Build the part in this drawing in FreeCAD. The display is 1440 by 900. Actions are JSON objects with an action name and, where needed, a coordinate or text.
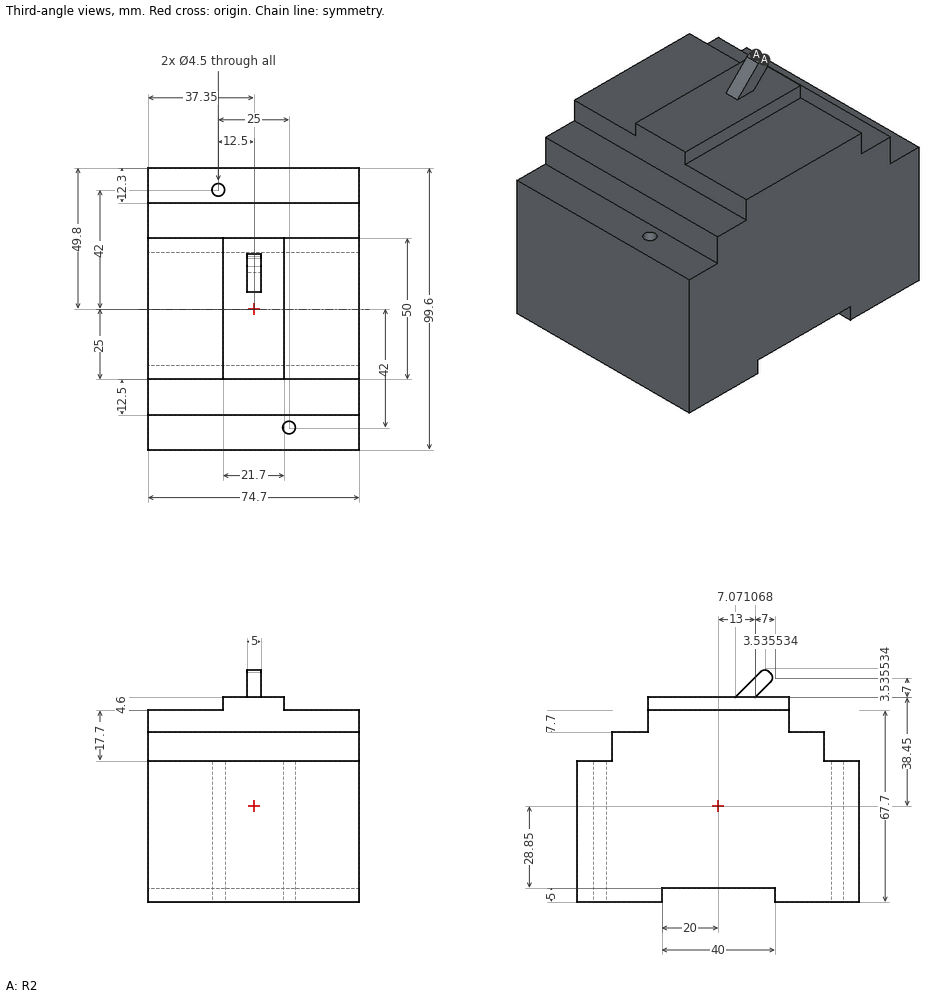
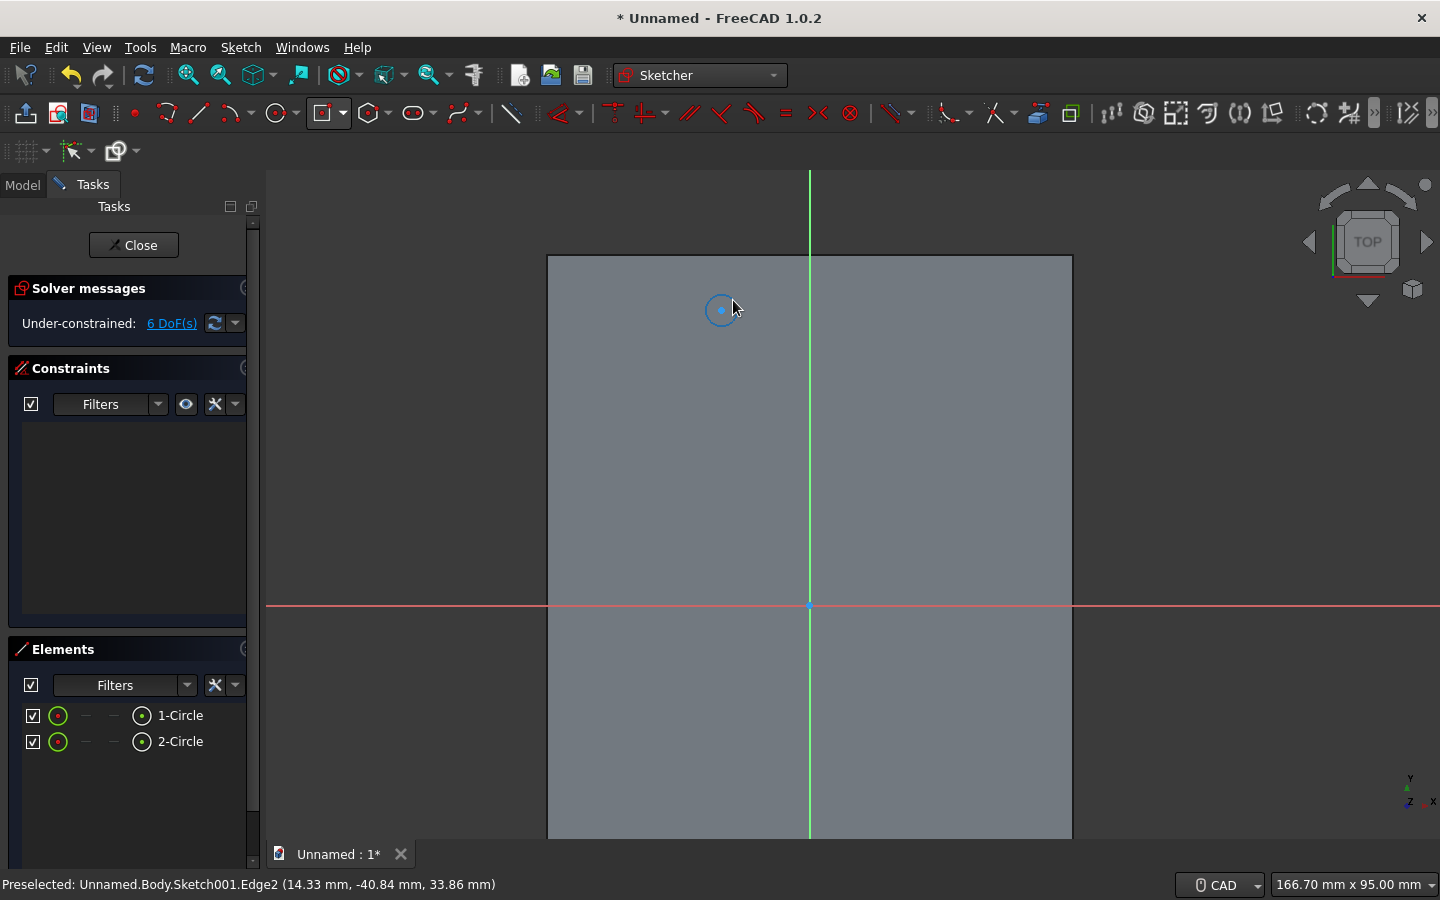
{"action": "left_click", "coordinate": [733, 299]}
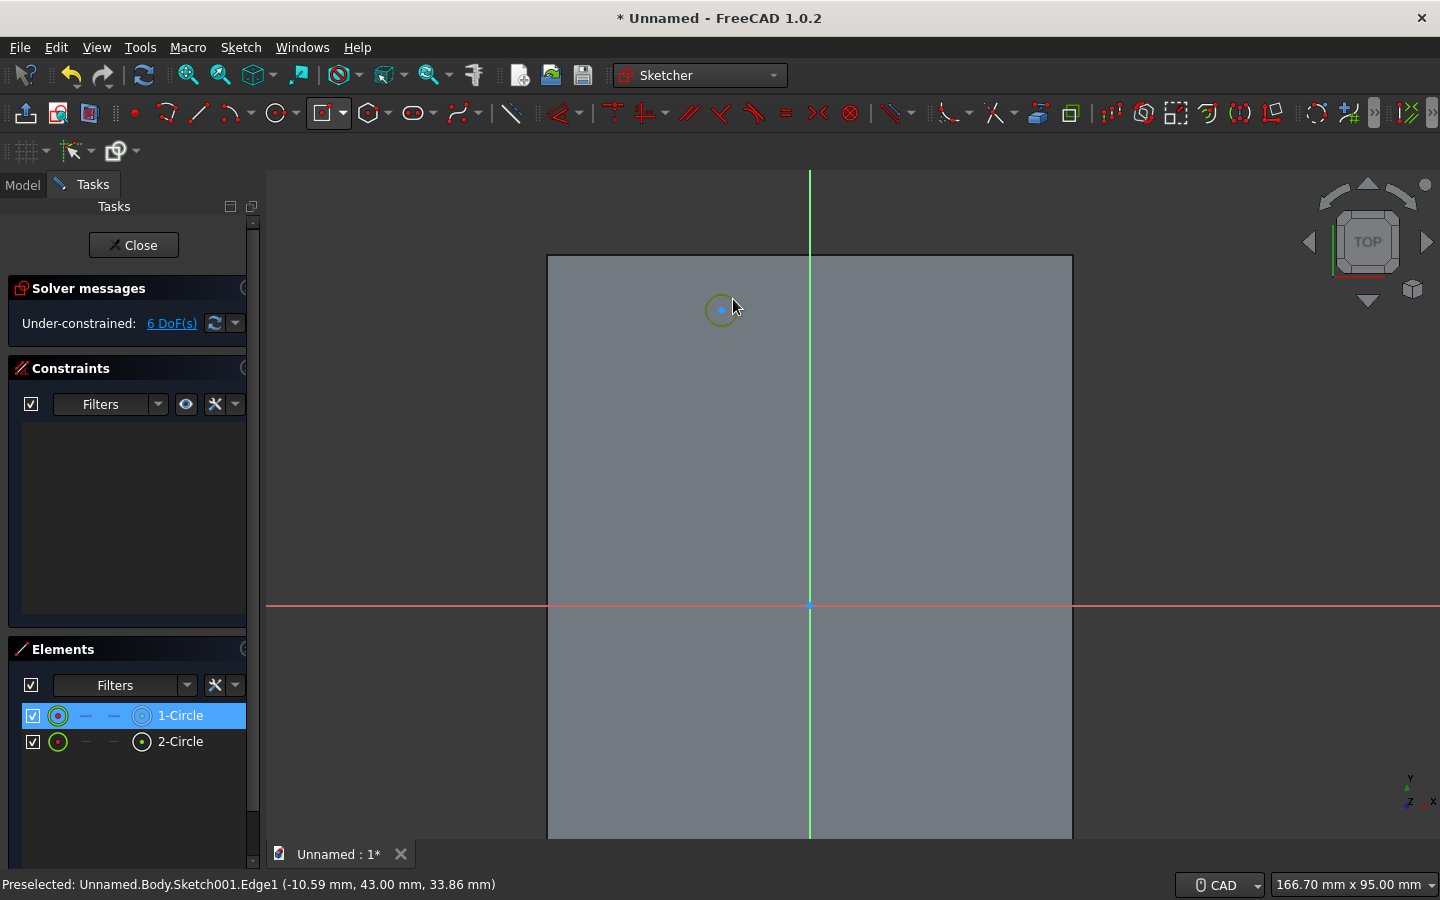
{"action": "scroll", "coordinate": [733, 299], "scroll_direction": "down", "scroll_amount": 2}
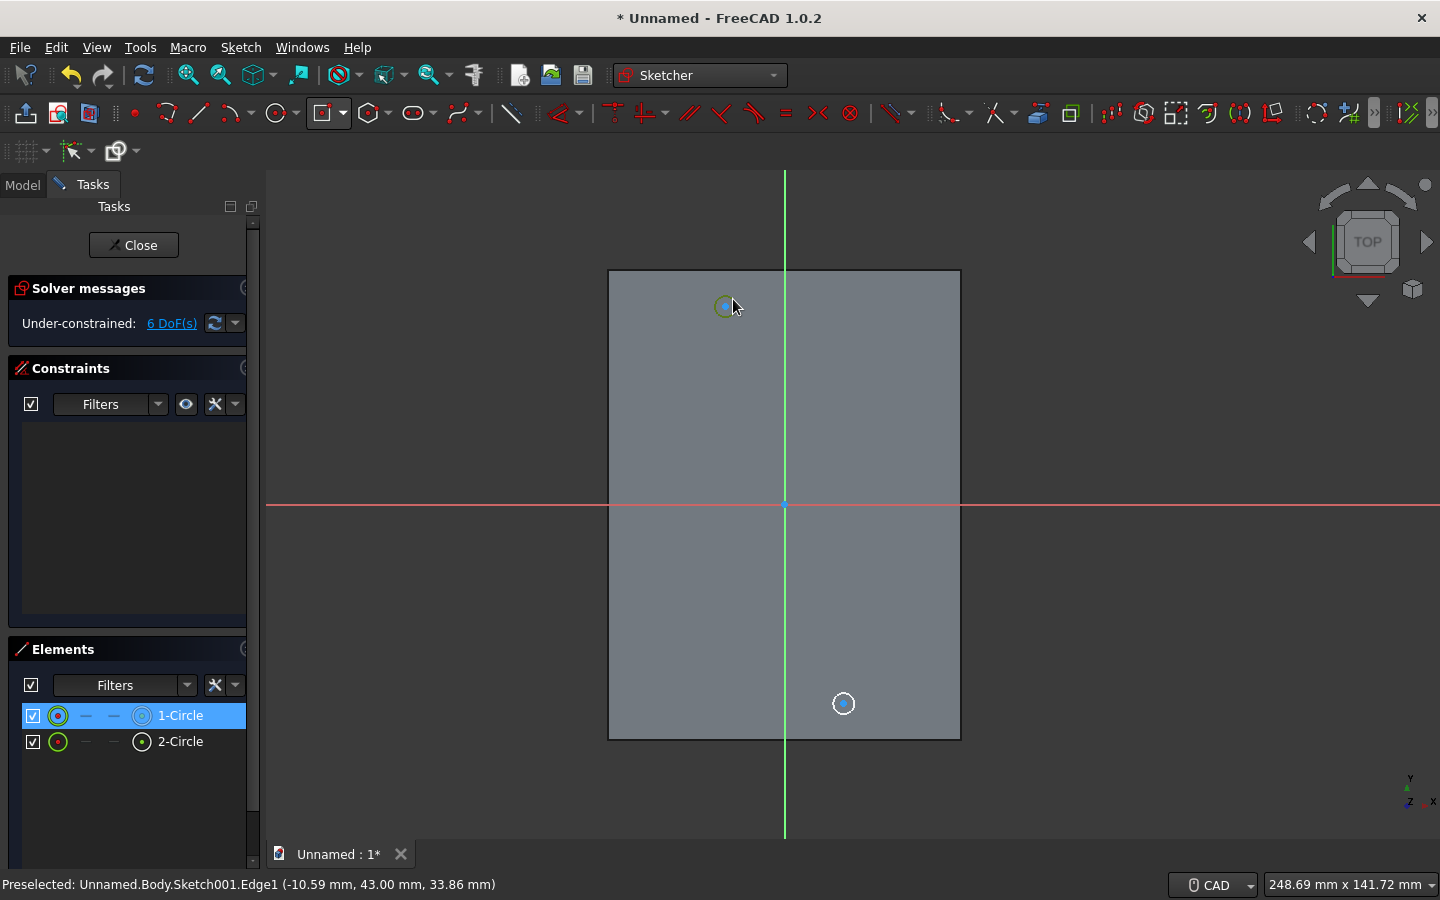
{"action": "scroll", "coordinate": [851, 696], "scroll_direction": "up", "scroll_amount": 2}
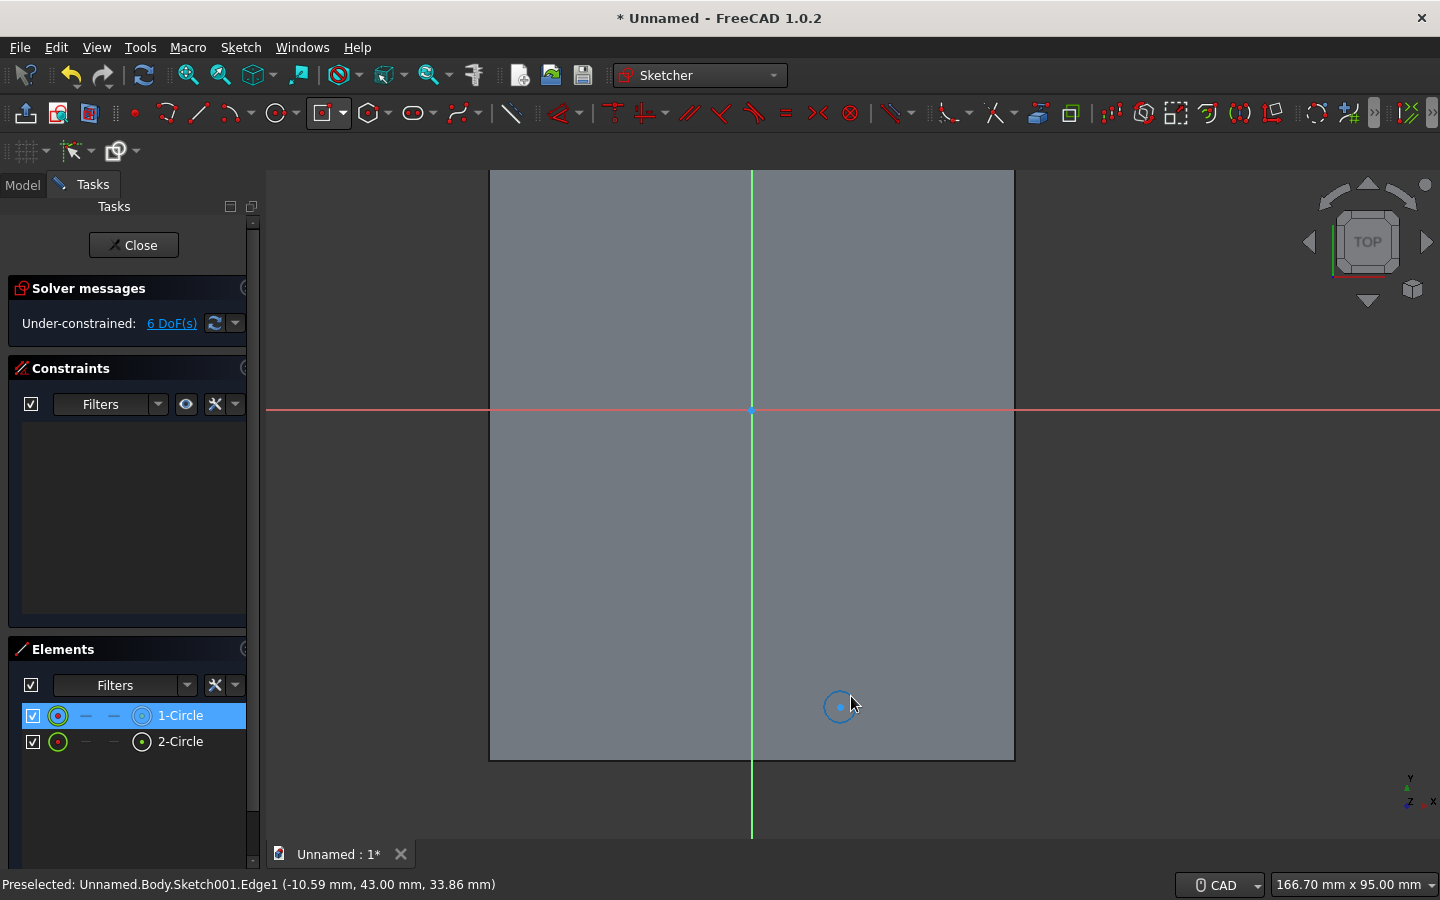
{"action": "left_click", "coordinate": [851, 696]}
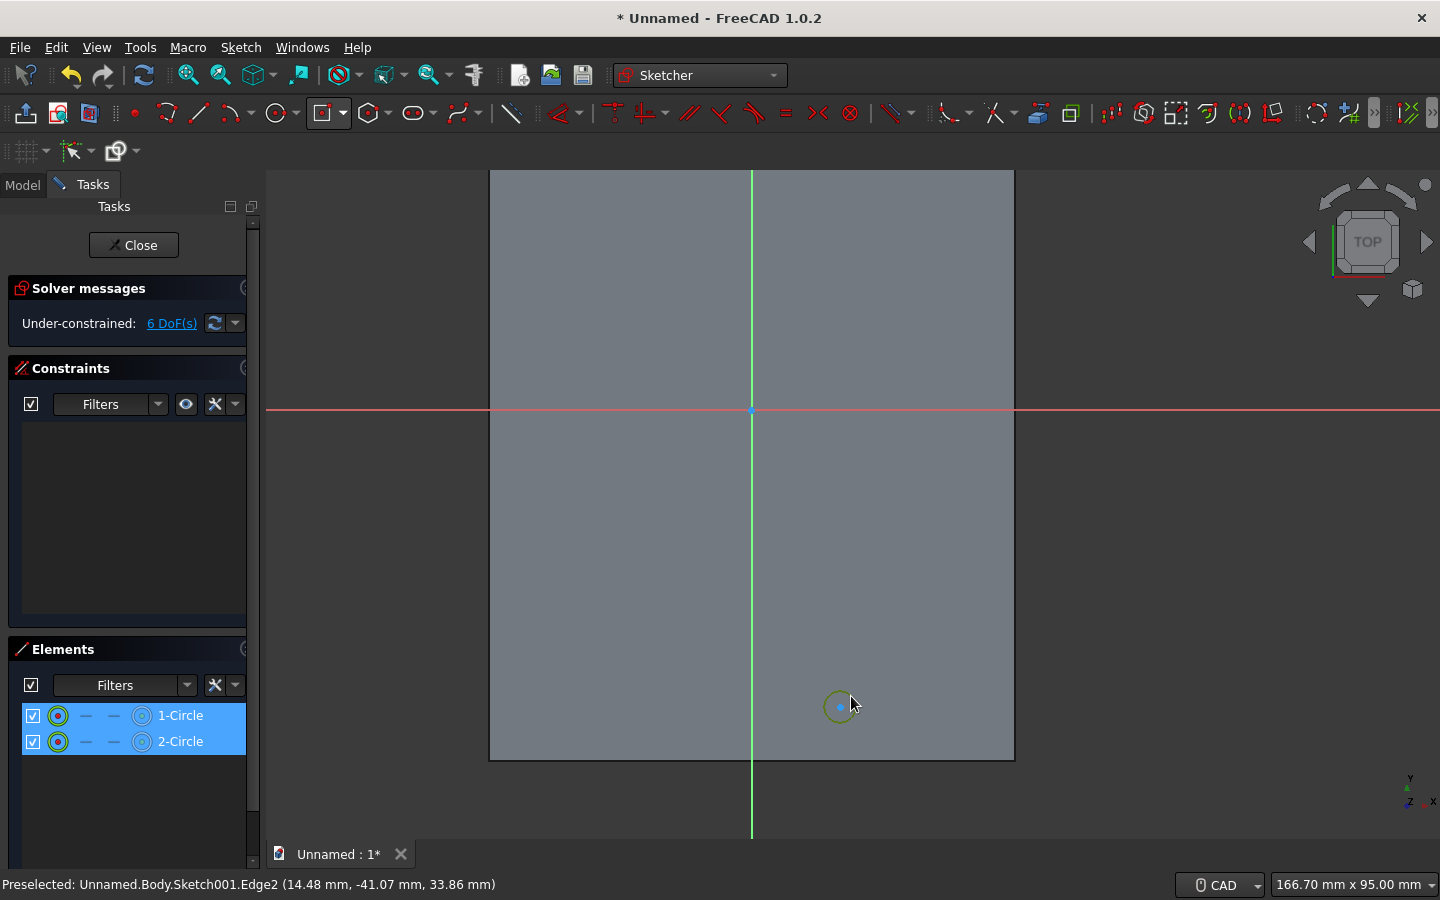
{"action": "left_click", "coordinate": [786, 114]}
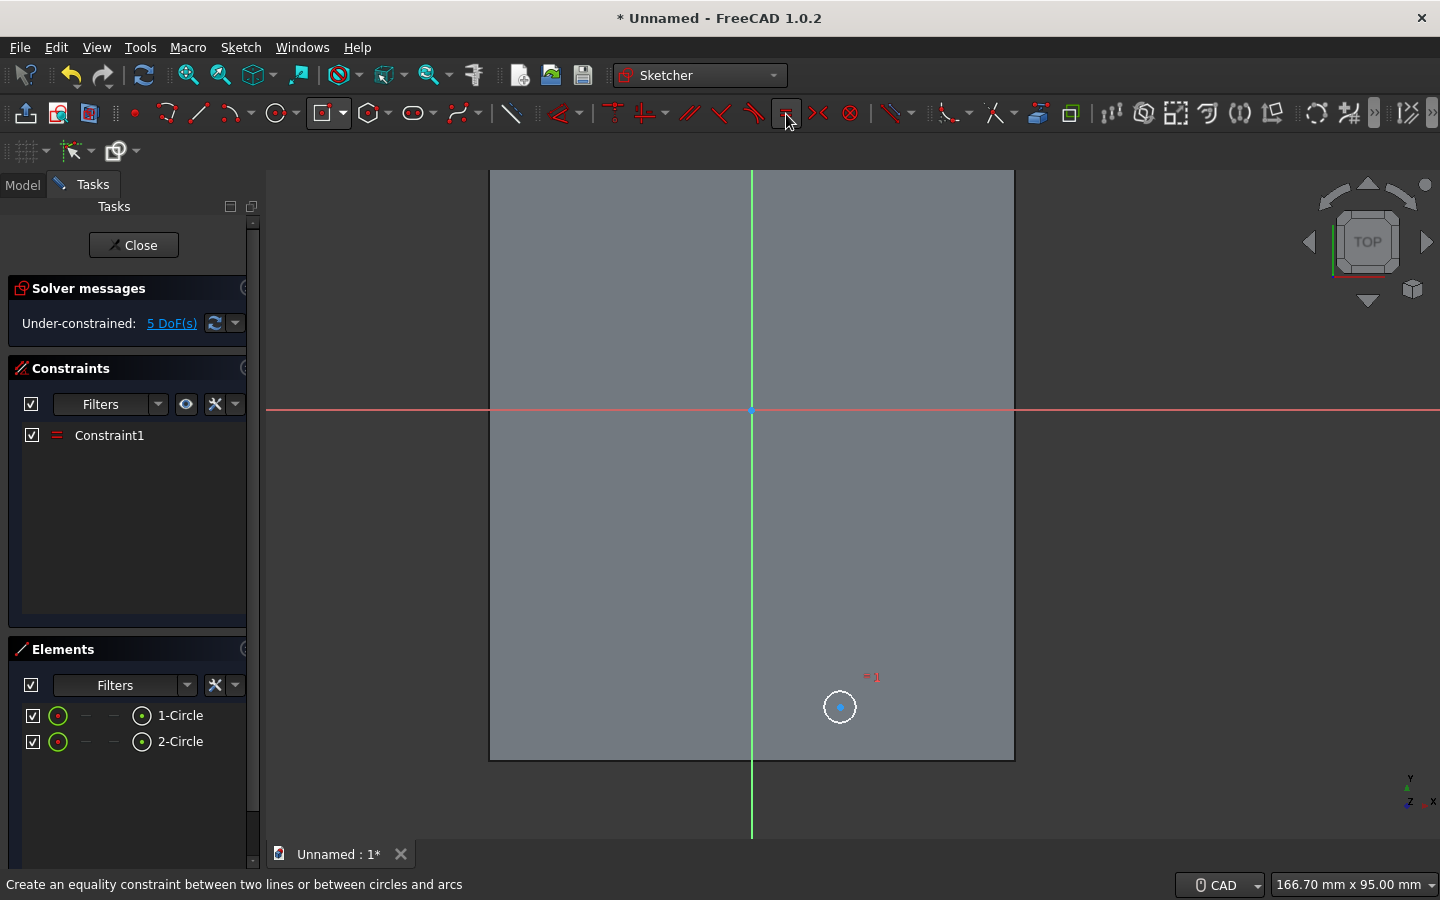
{"action": "left_click", "coordinate": [558, 114]}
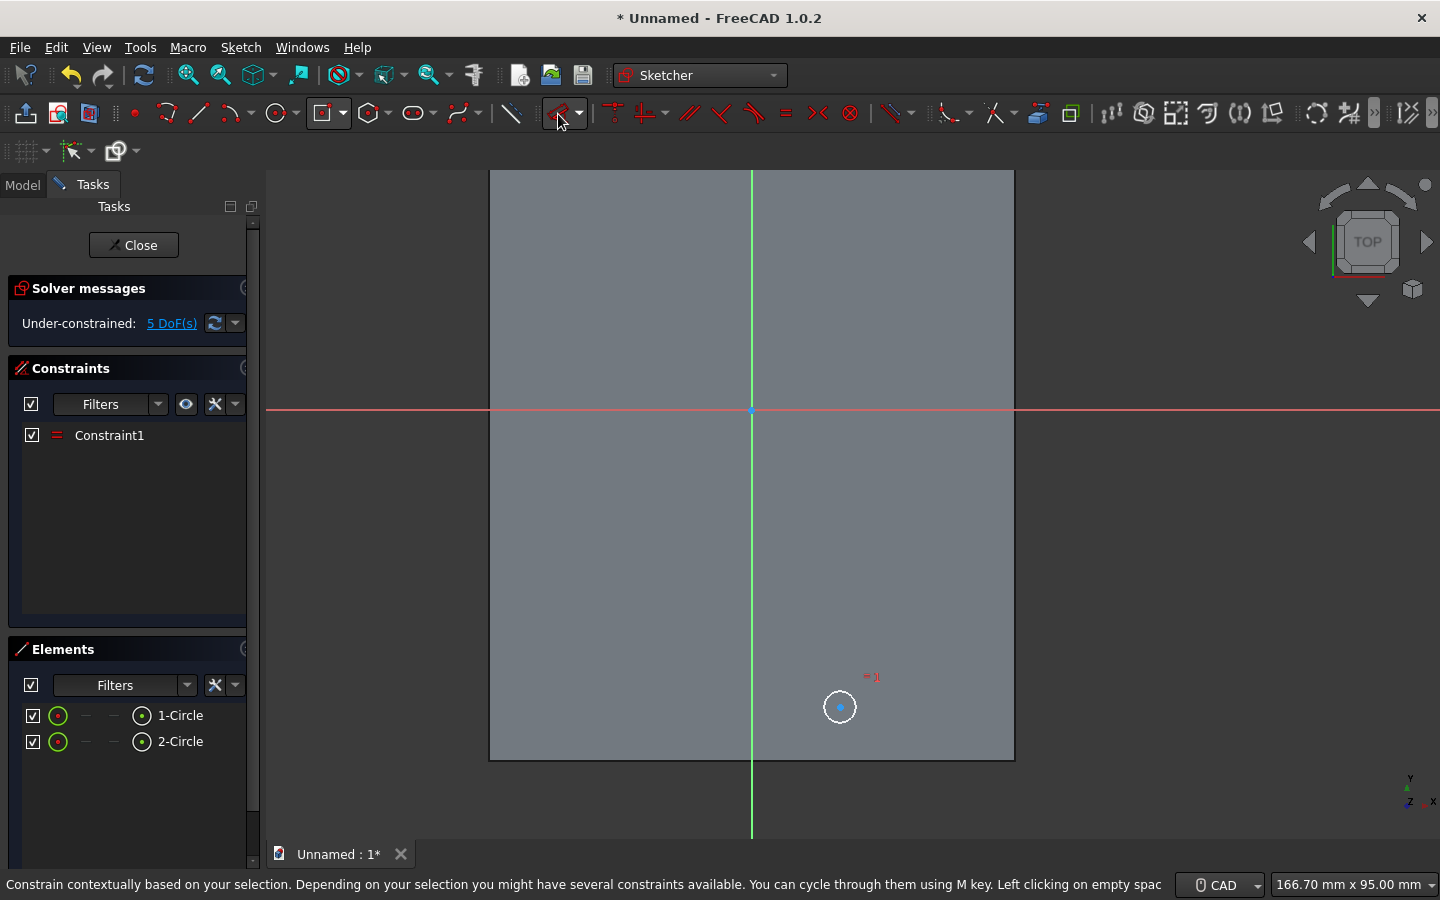
{"action": "scroll", "coordinate": [851, 696], "scroll_direction": "down", "scroll_amount": 2}